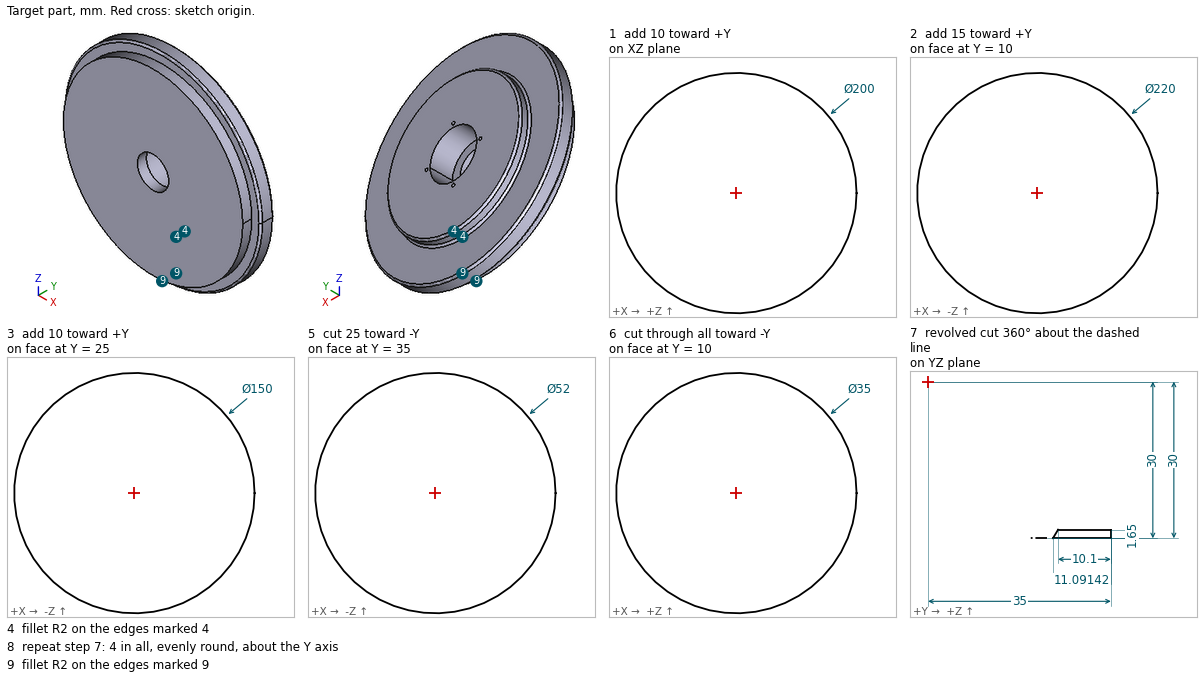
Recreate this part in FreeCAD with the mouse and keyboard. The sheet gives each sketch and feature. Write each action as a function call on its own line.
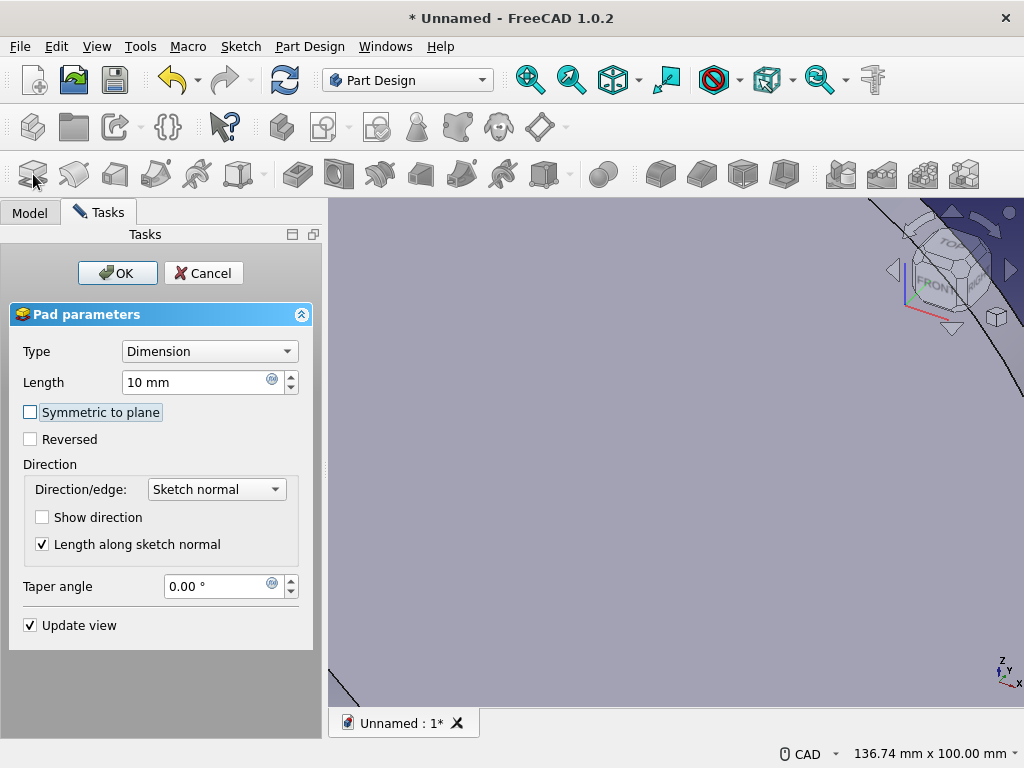
click(31, 439)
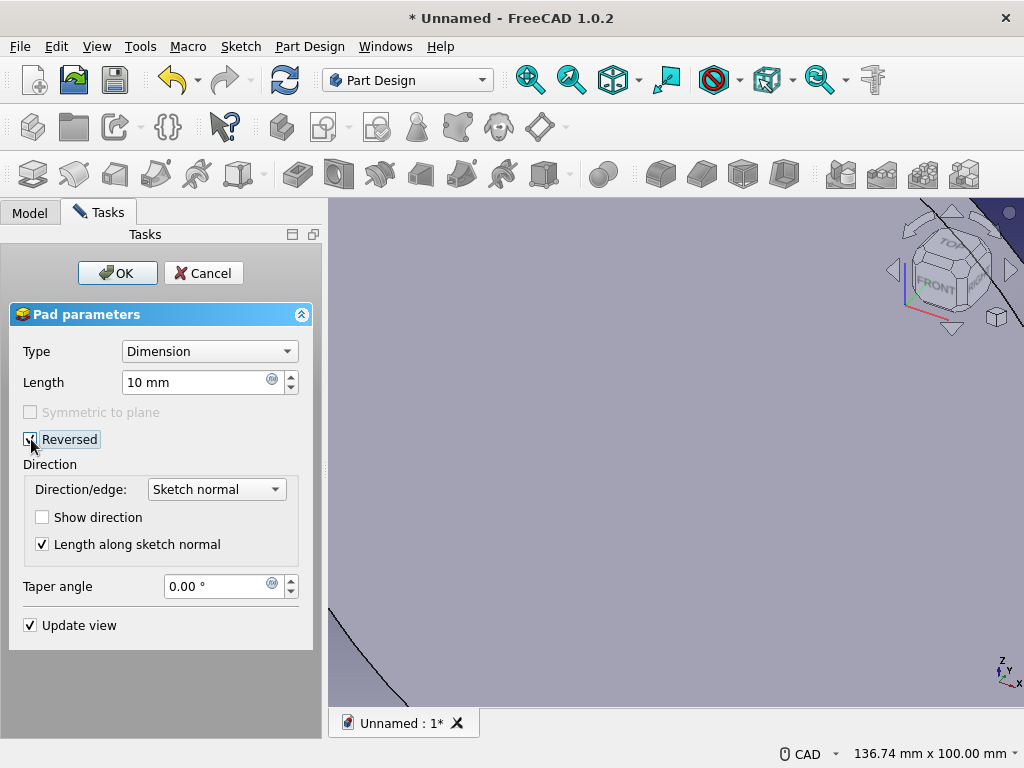
click(118, 273)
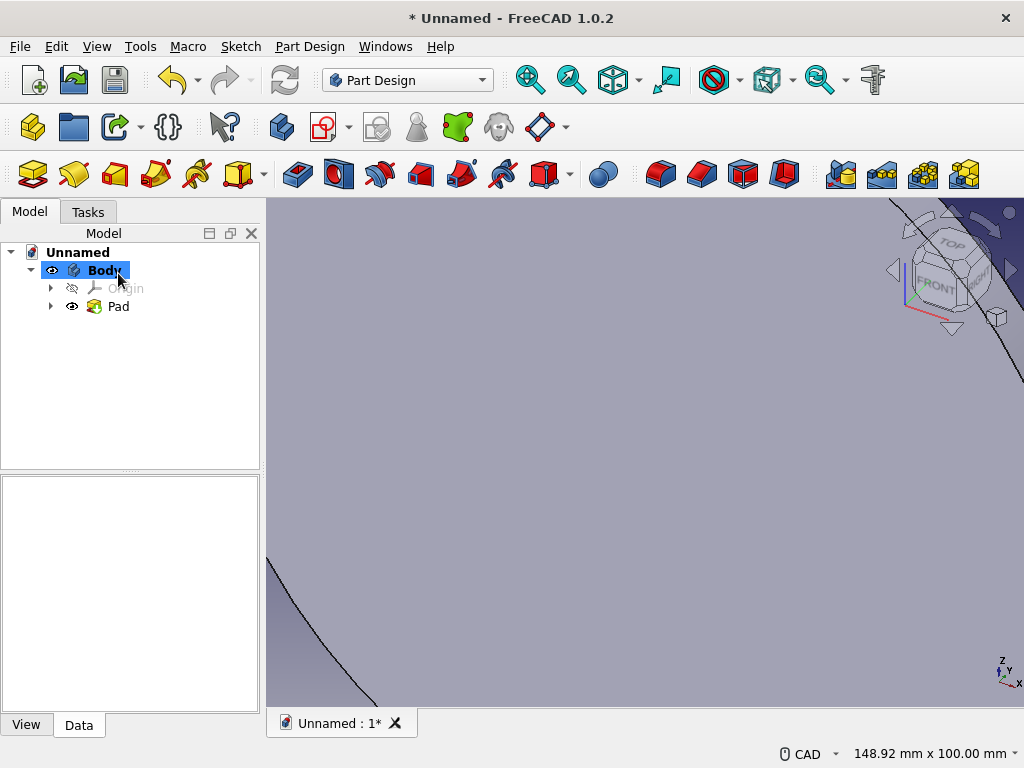
click(531, 80)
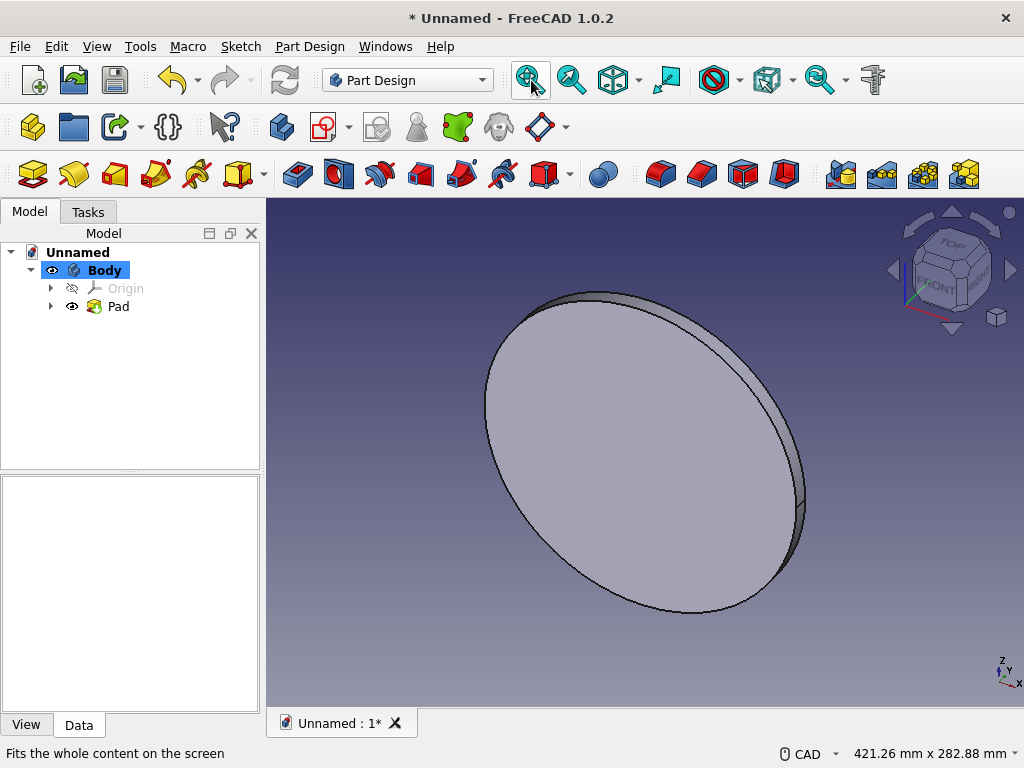
key(4)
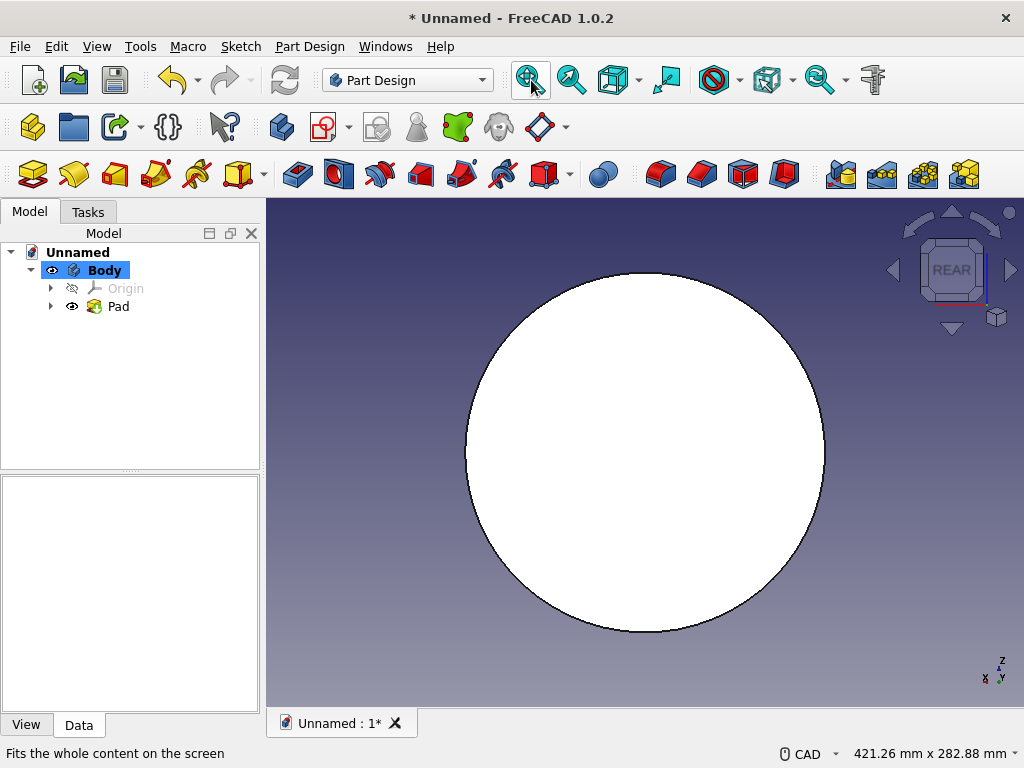
click(645, 451)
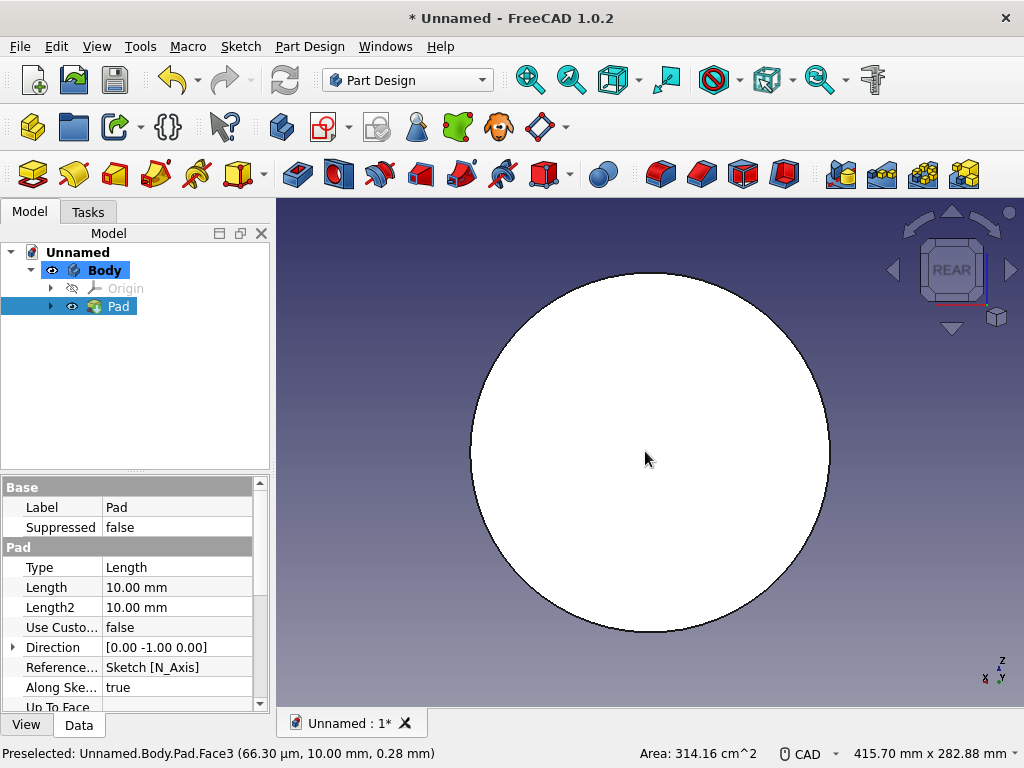
click(322, 128)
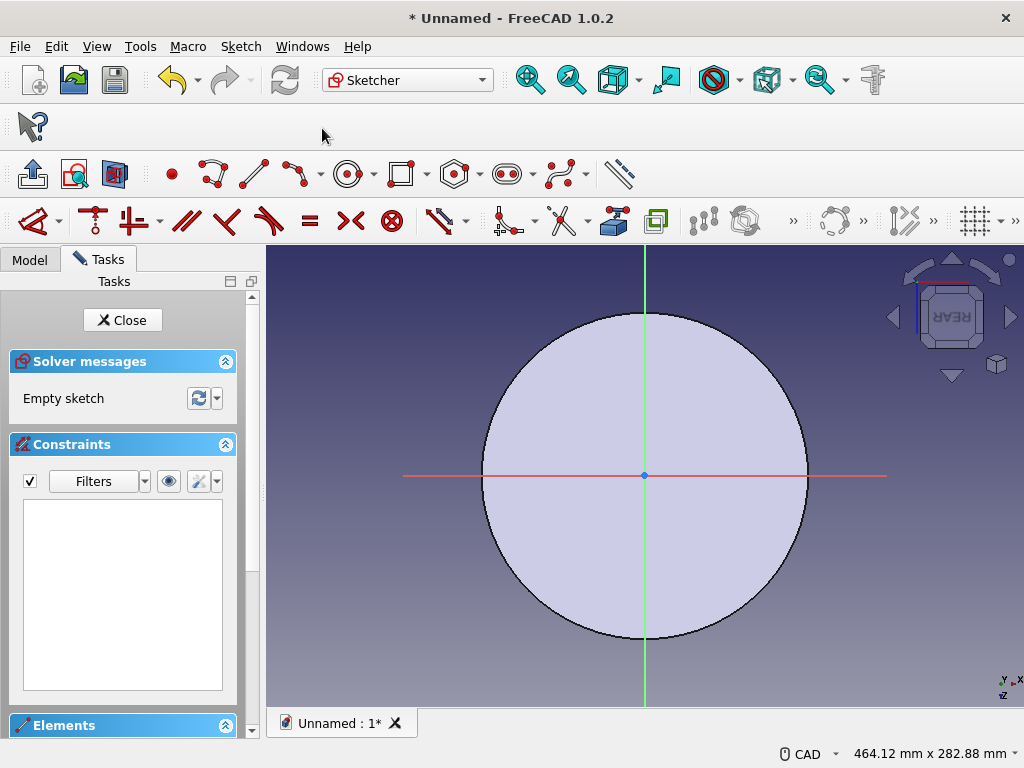
scroll(294, 476, down, 1)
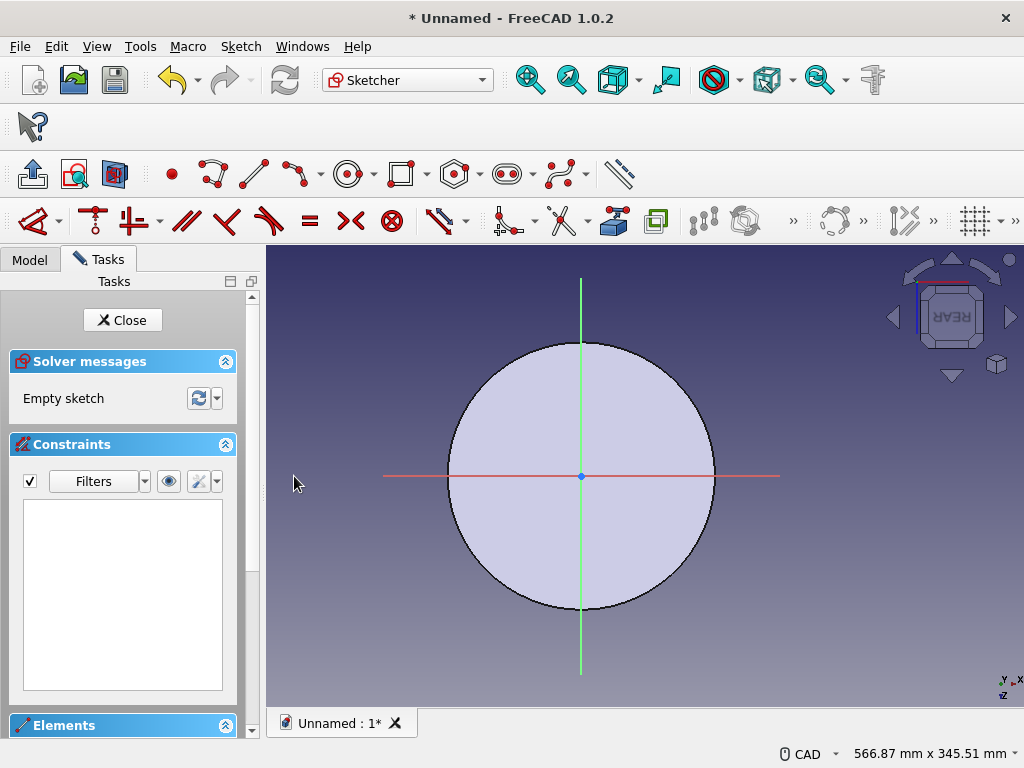
click(348, 174)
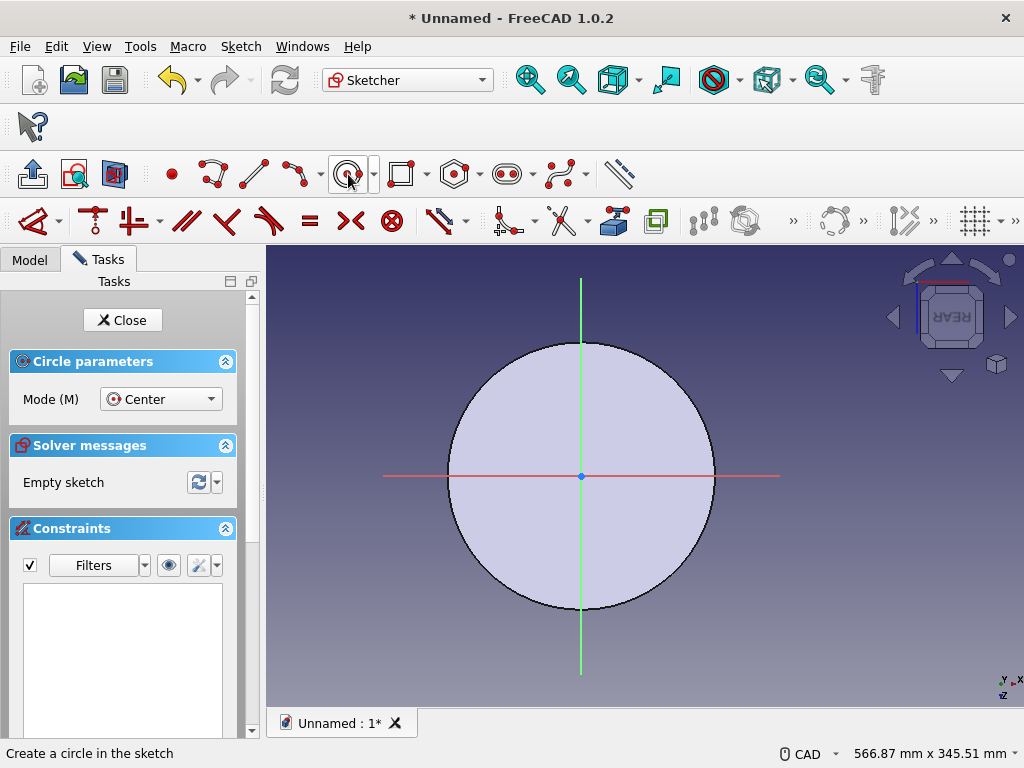
click(581, 476)
click(685, 372)
key(Escape)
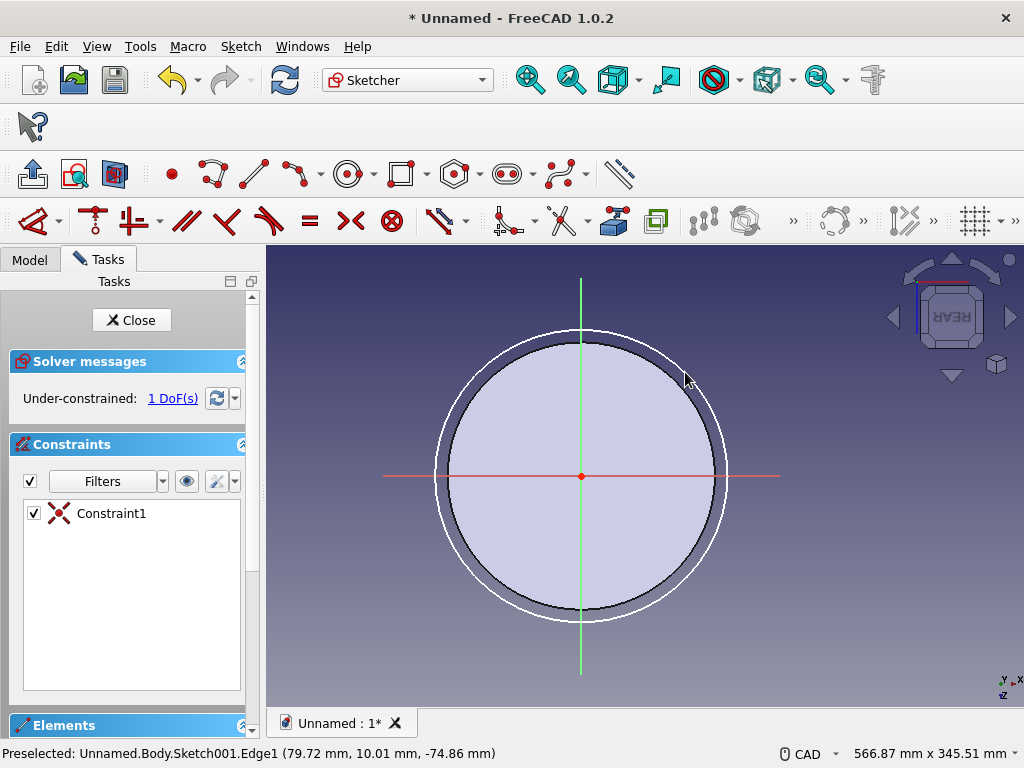
click(32, 222)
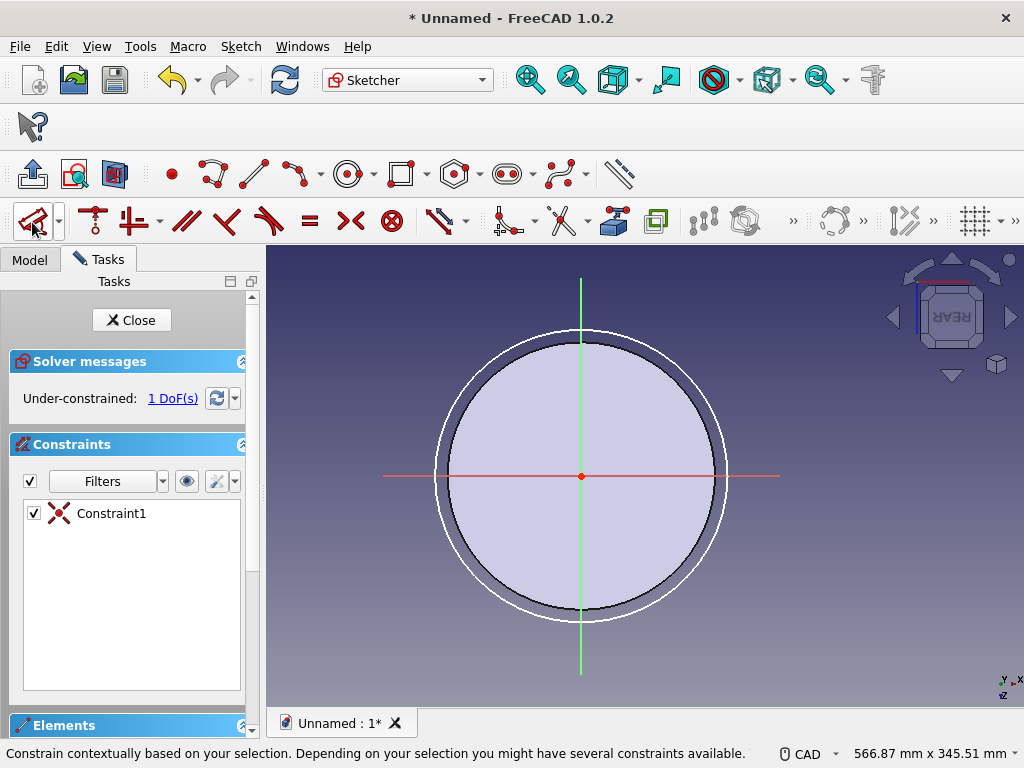
click(684, 372)
click(706, 349)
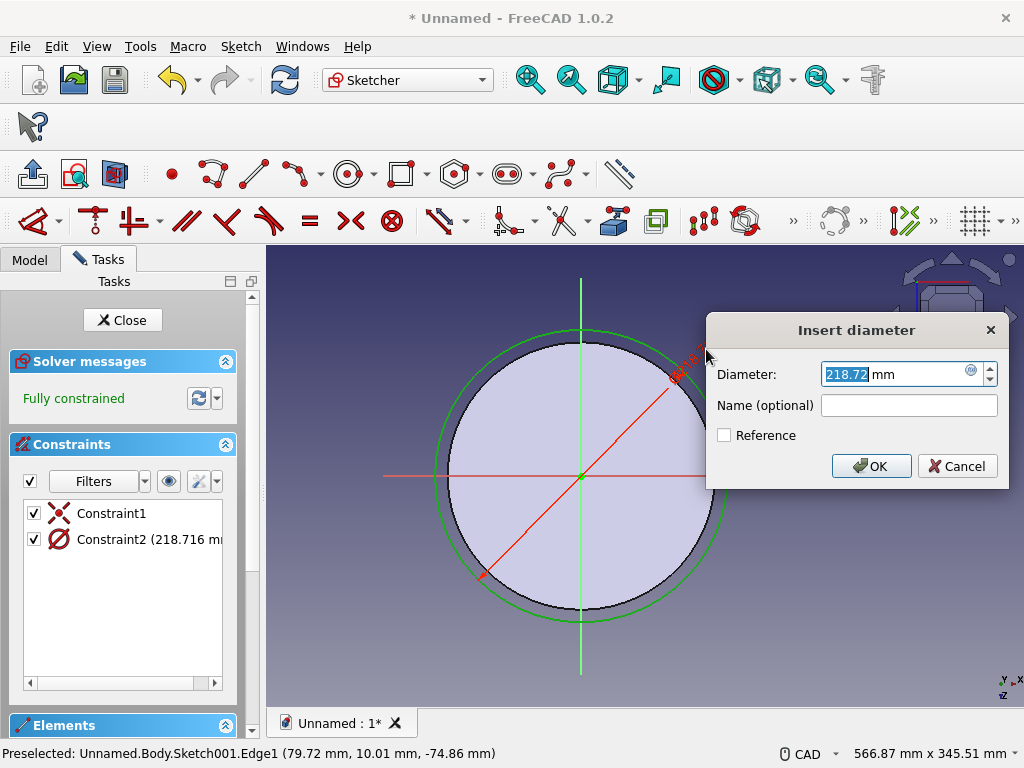
text(220)
key(Return)
key(Escape)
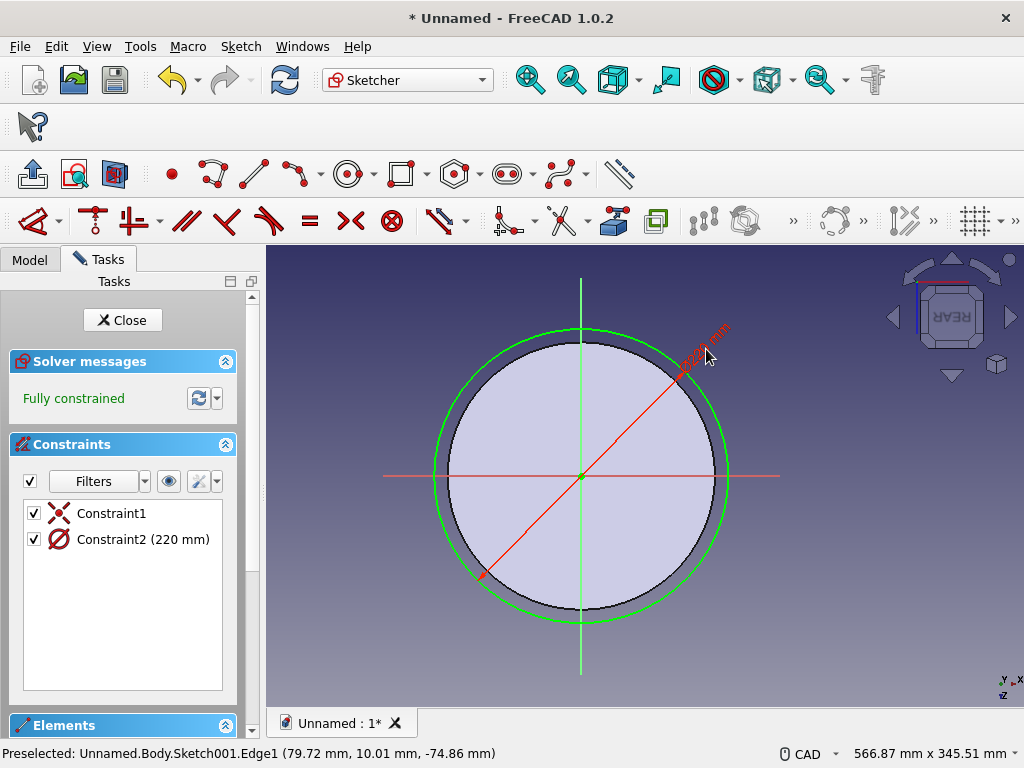
click(123, 320)